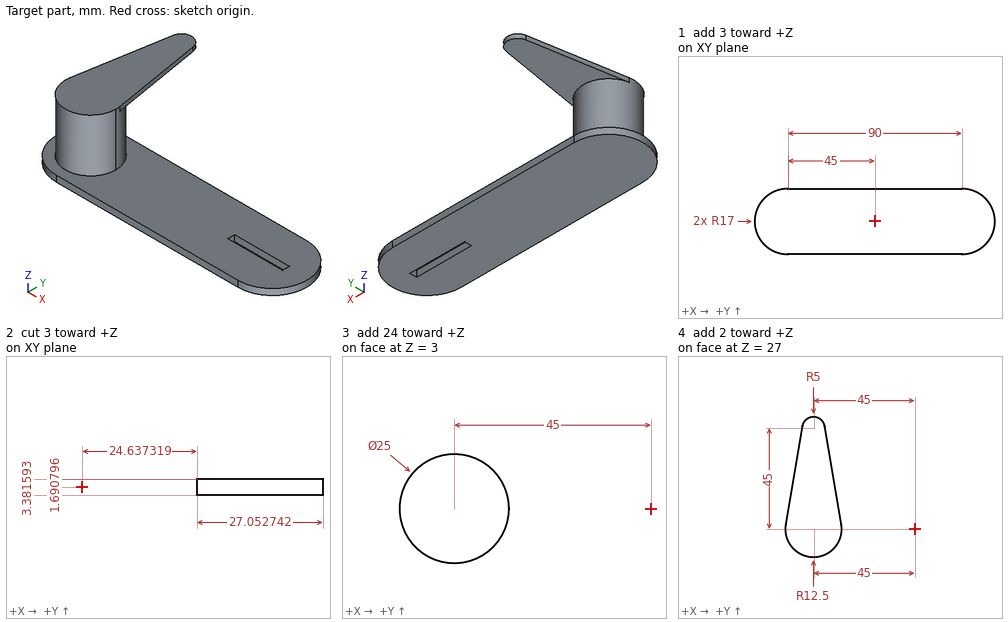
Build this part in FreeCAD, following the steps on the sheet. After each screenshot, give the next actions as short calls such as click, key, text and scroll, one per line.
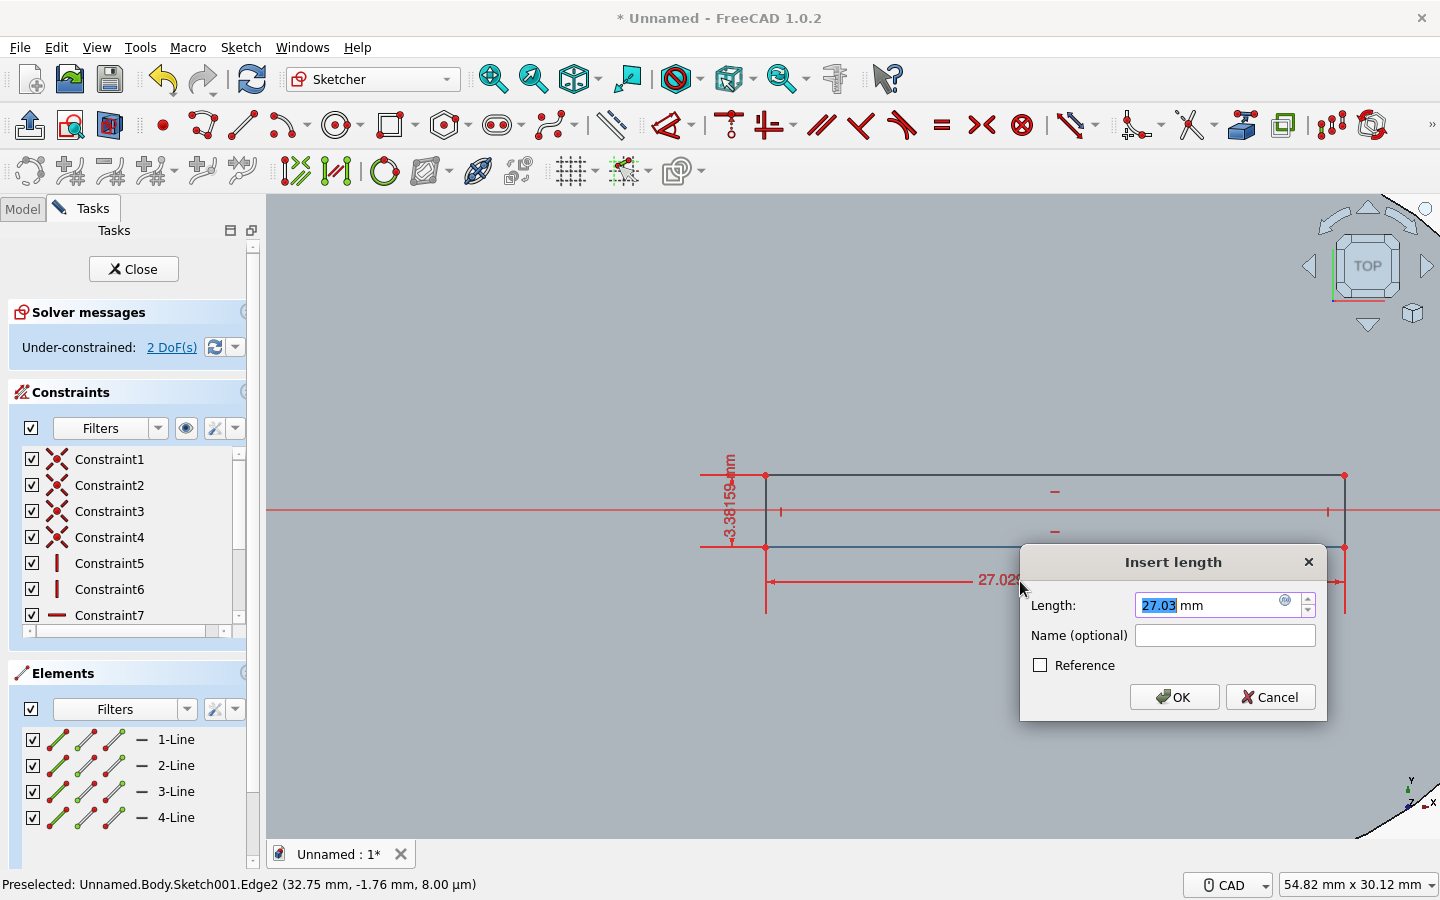
text(27.052742)
key(Return)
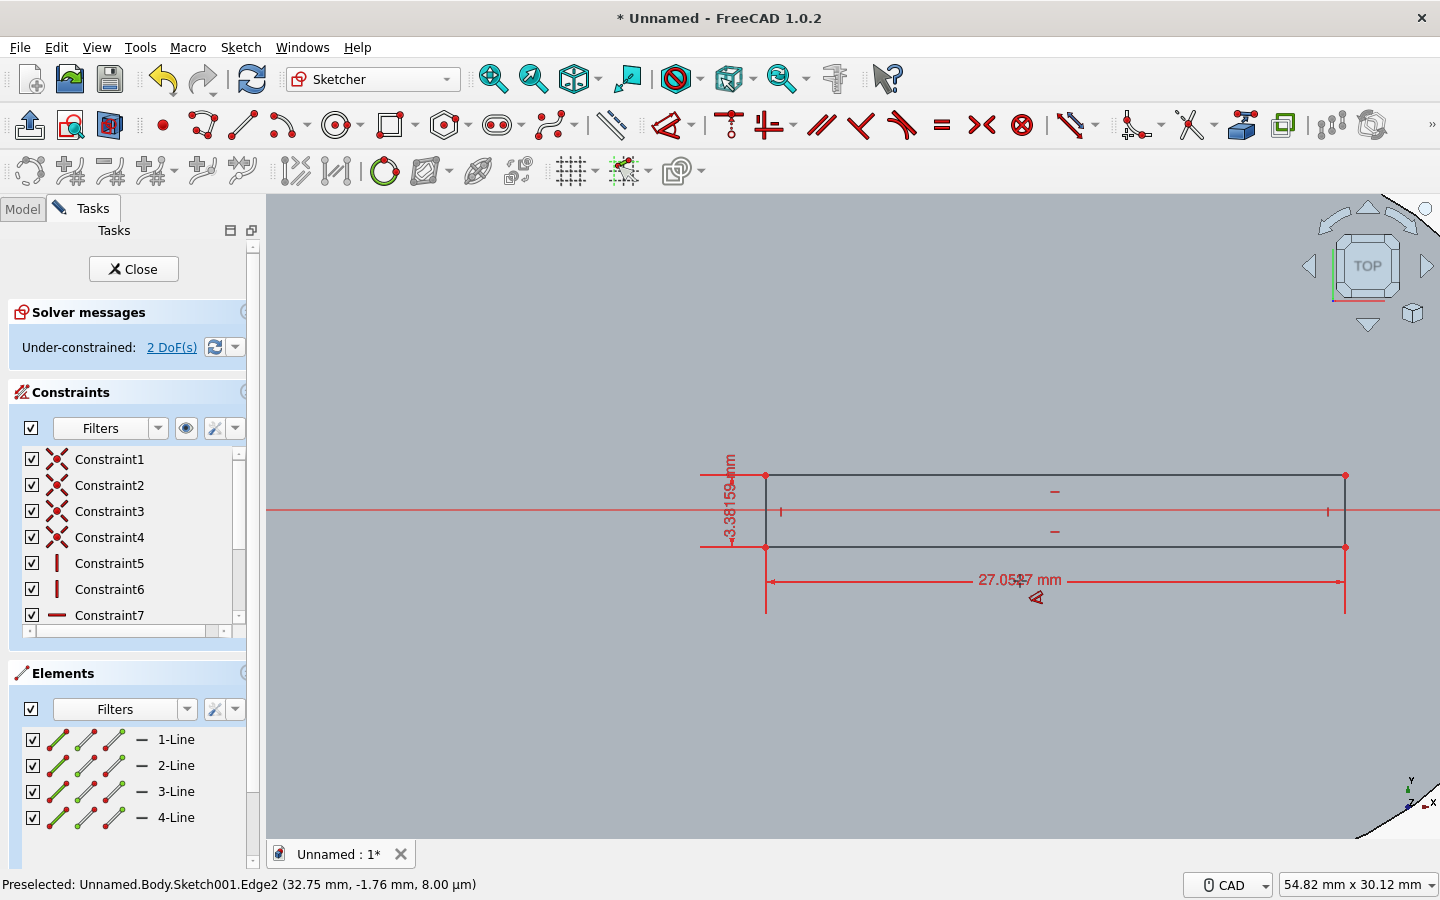
click(766, 475)
click(824, 492)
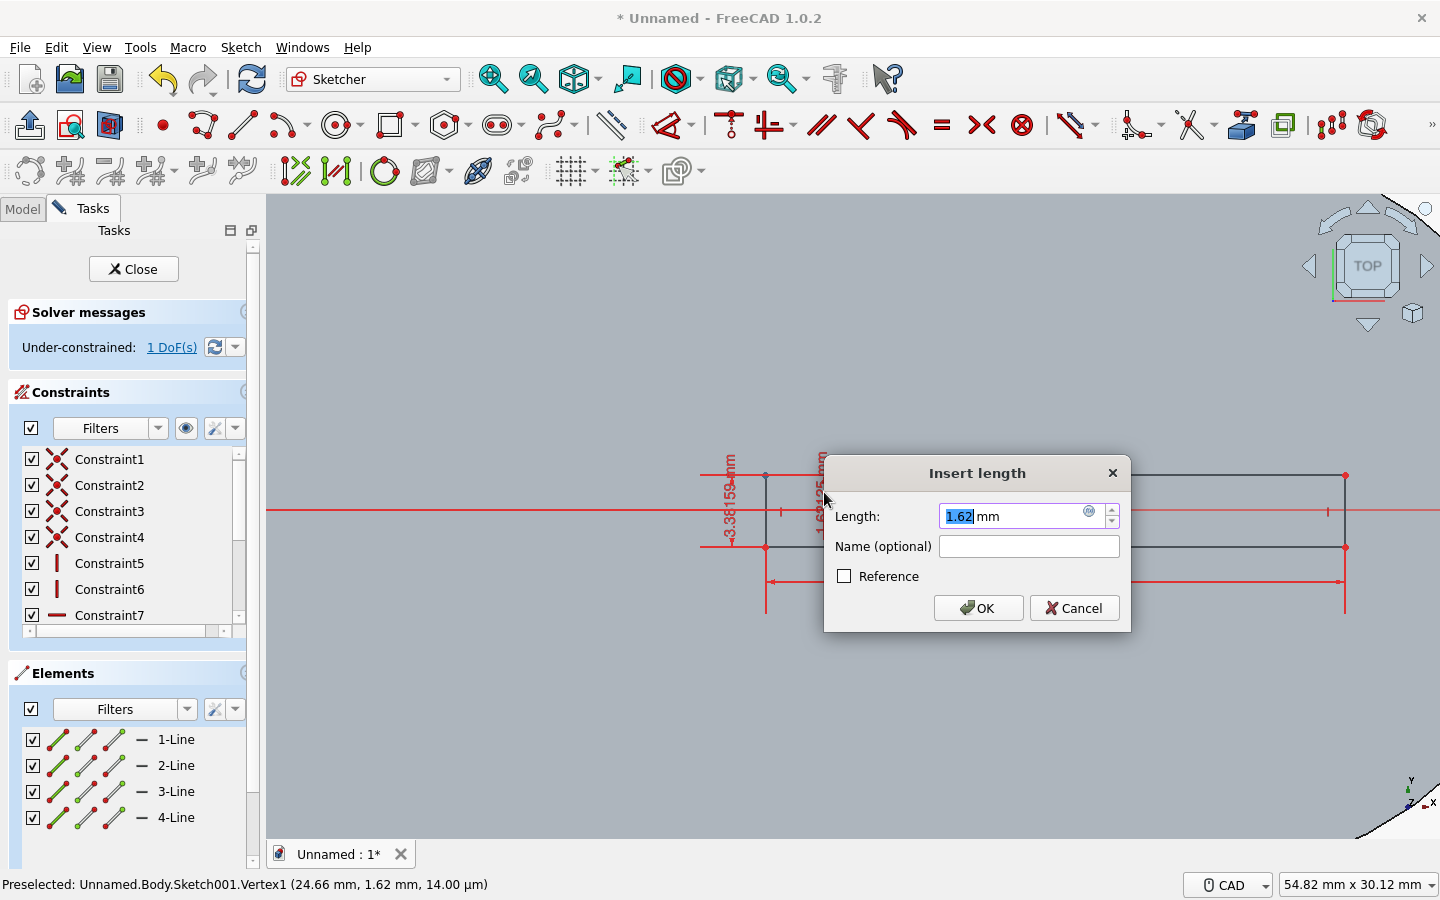
text(1.690796)
key(Return)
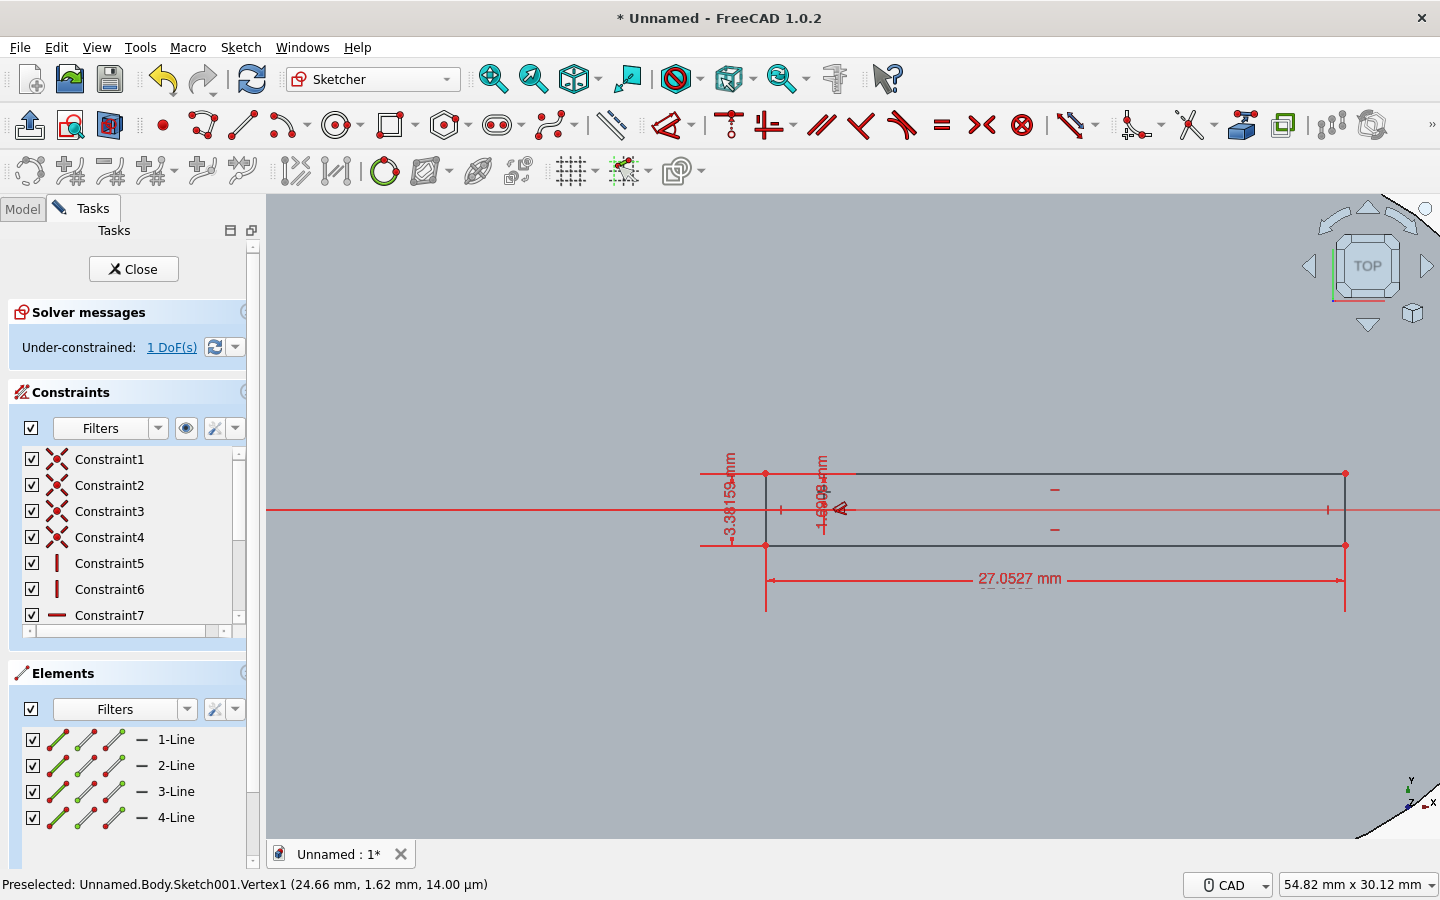
click(766, 474)
click(530, 440)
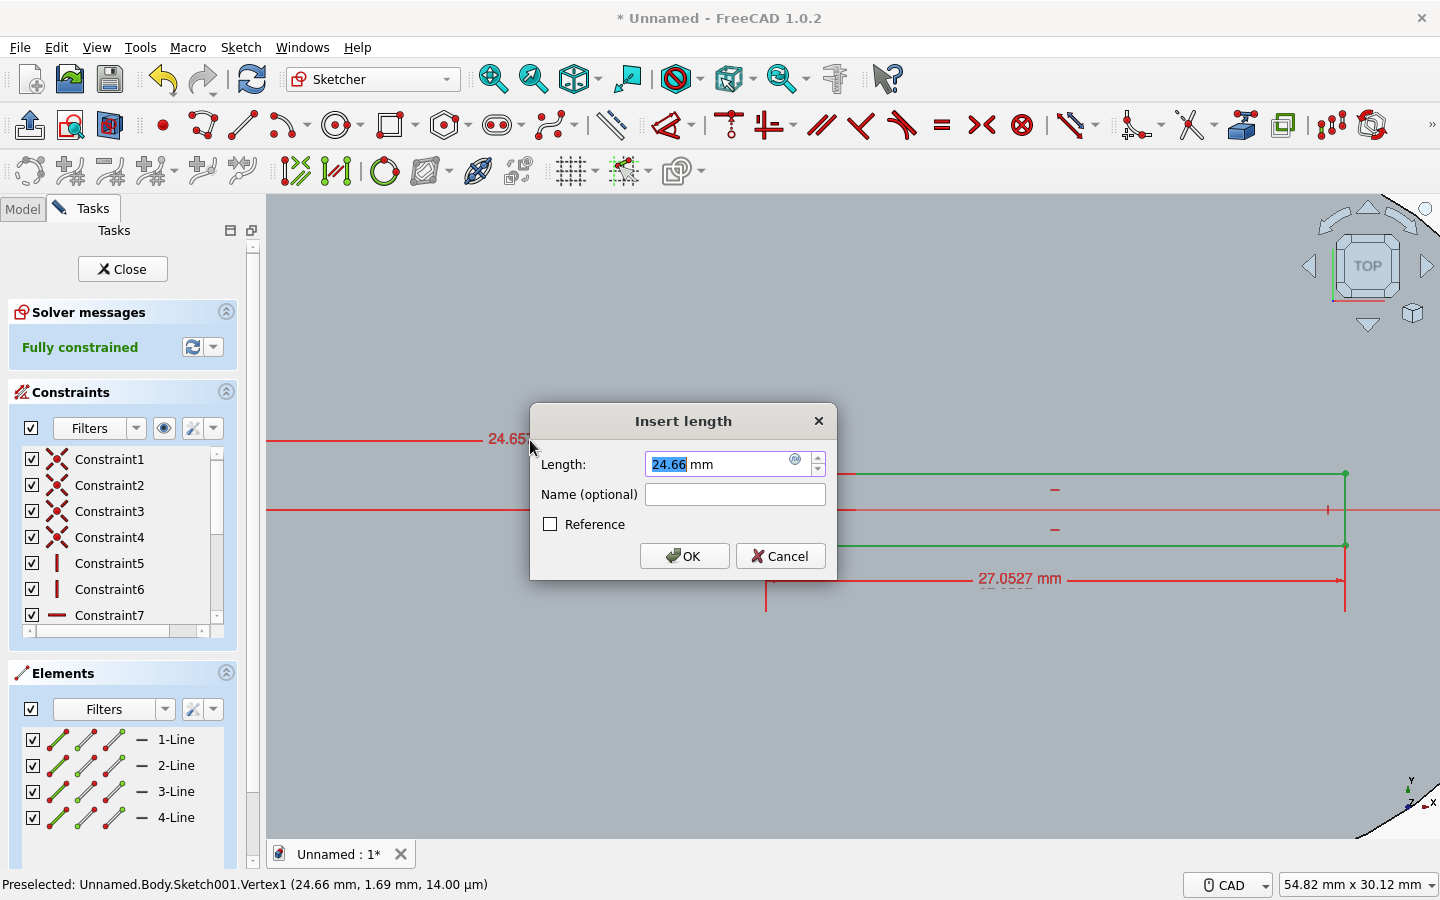
text(24.637319)
key(Return)
key(Escape)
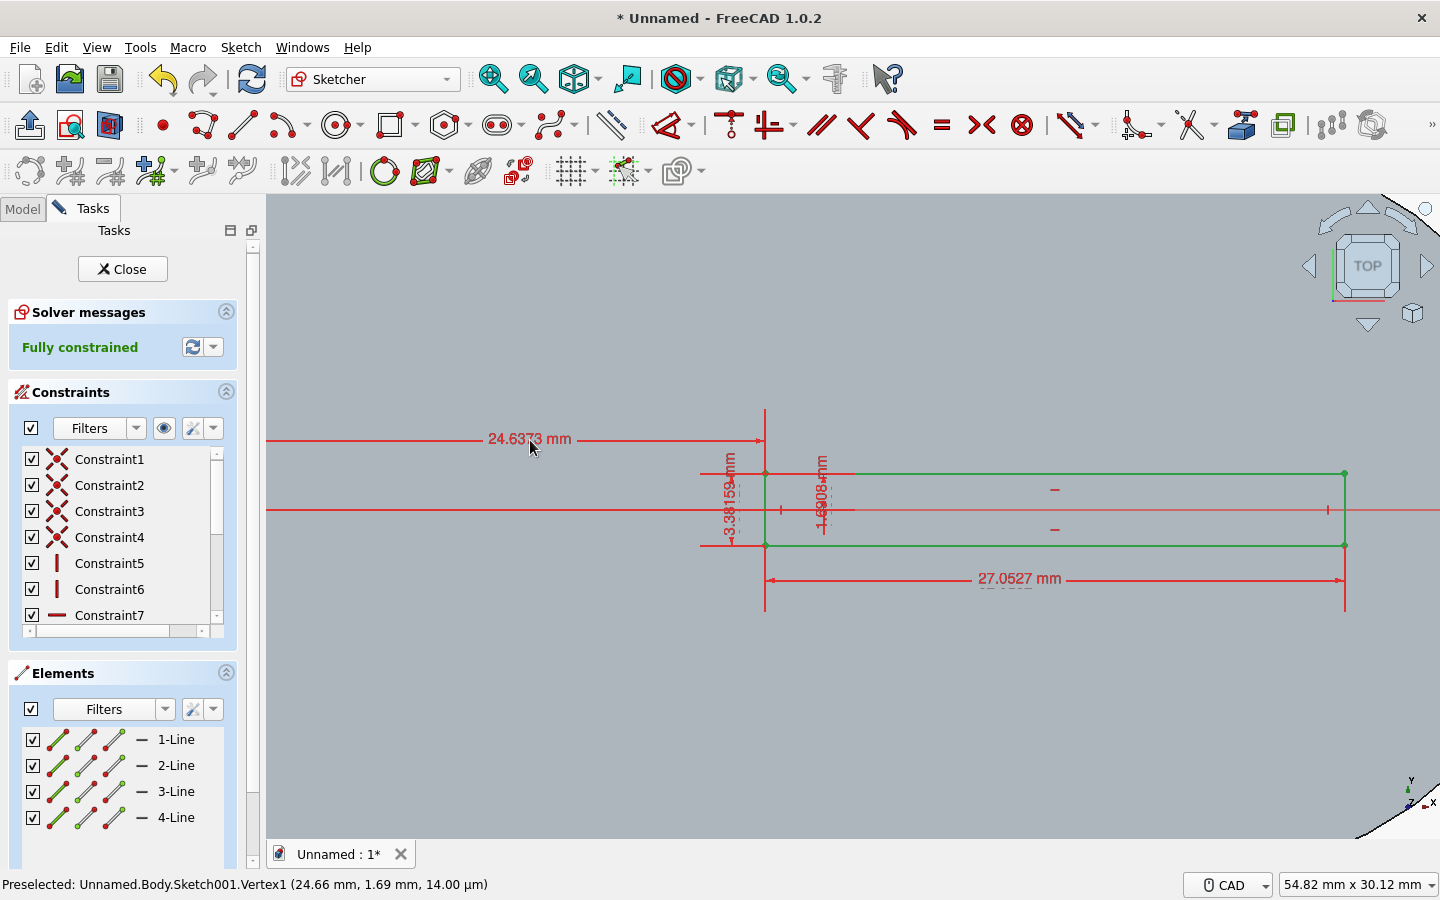
click(123, 269)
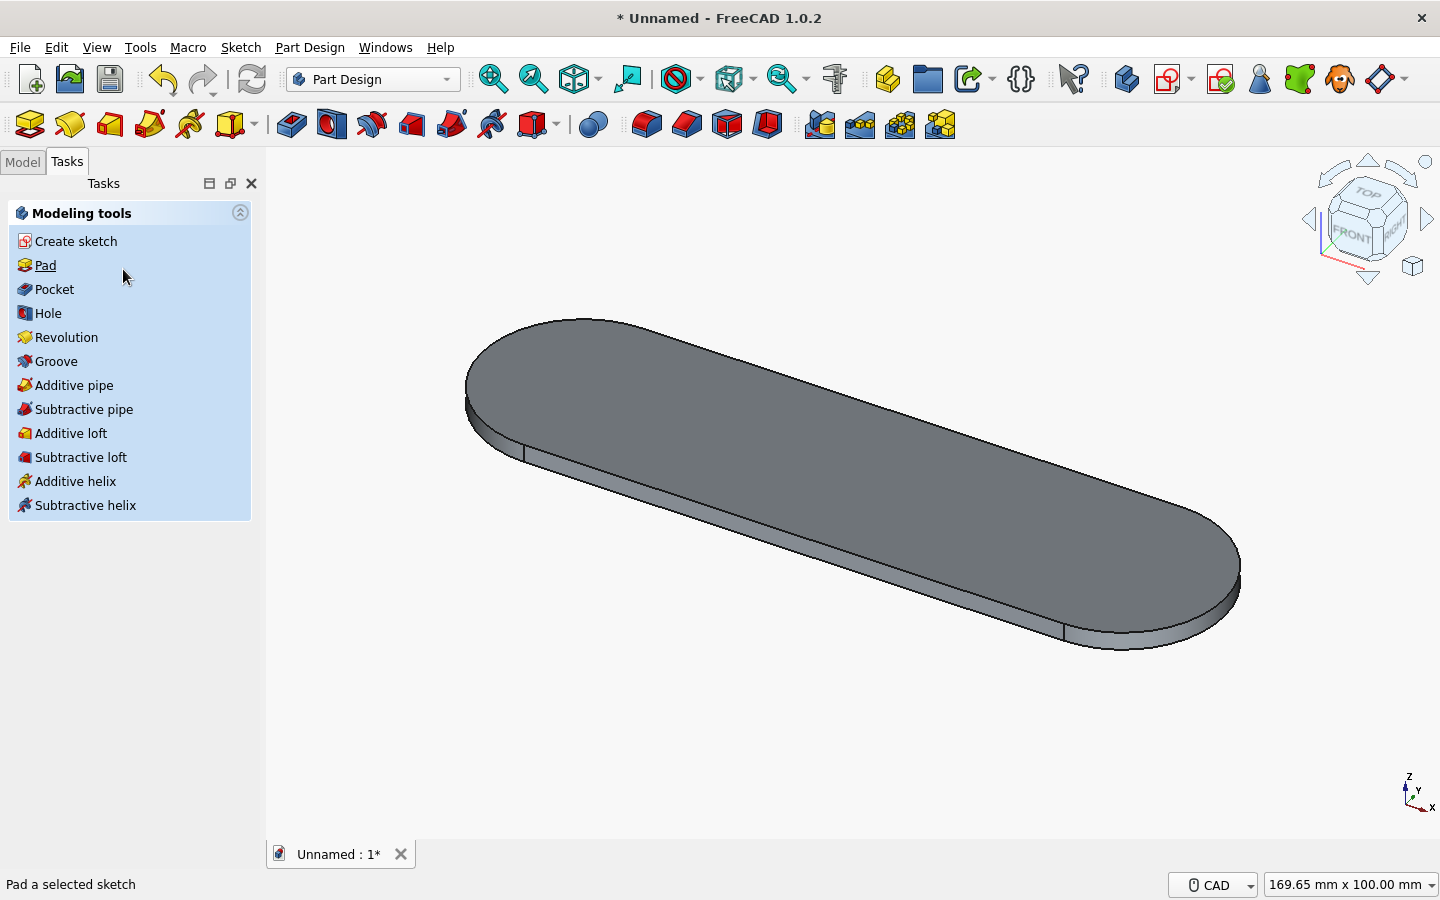
click(292, 124)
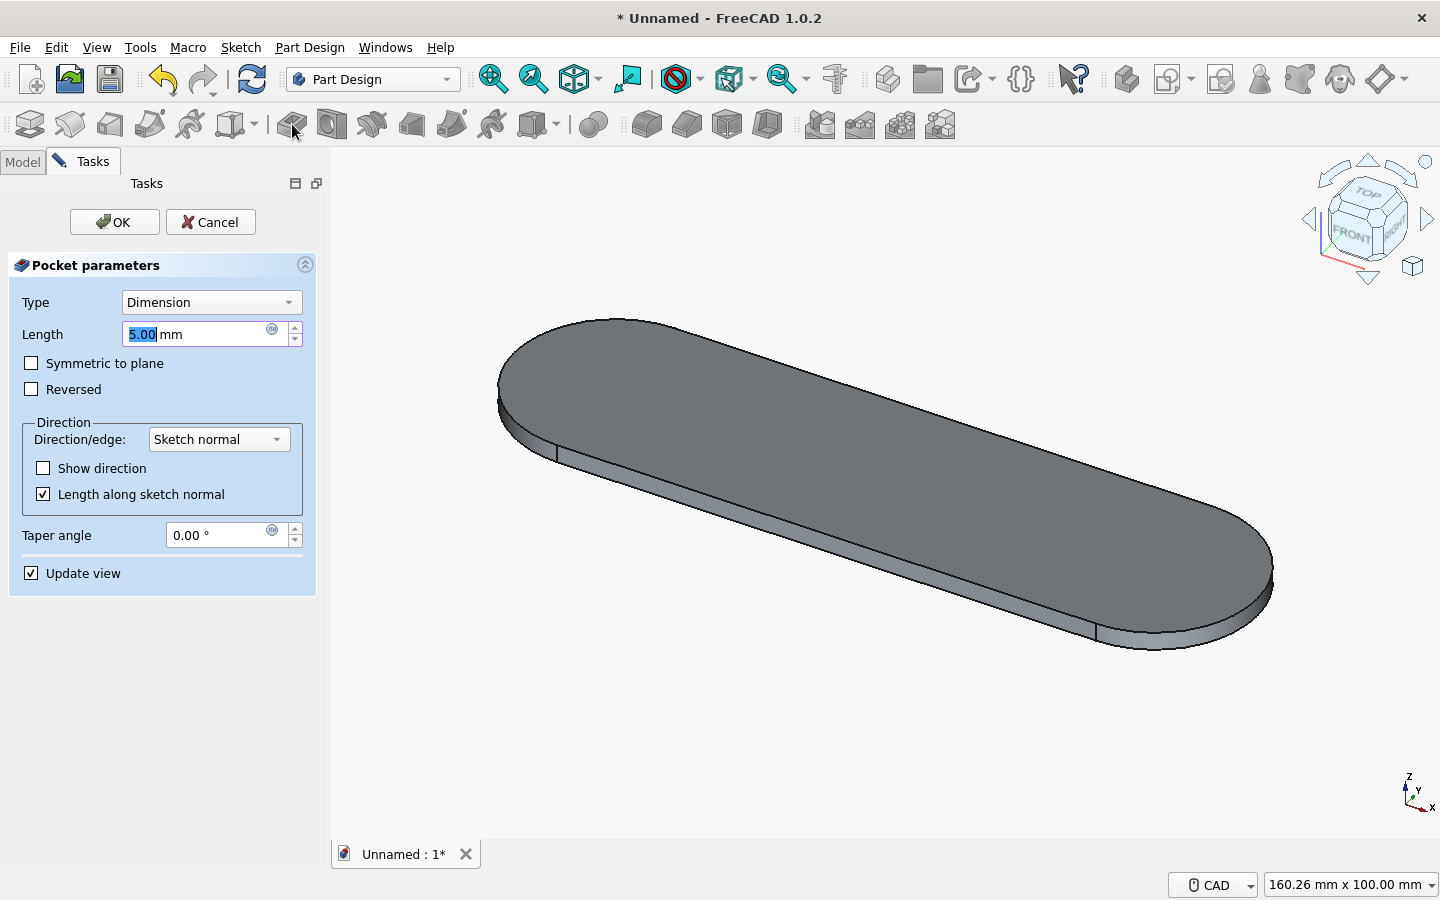
text(3)
key(Tab)